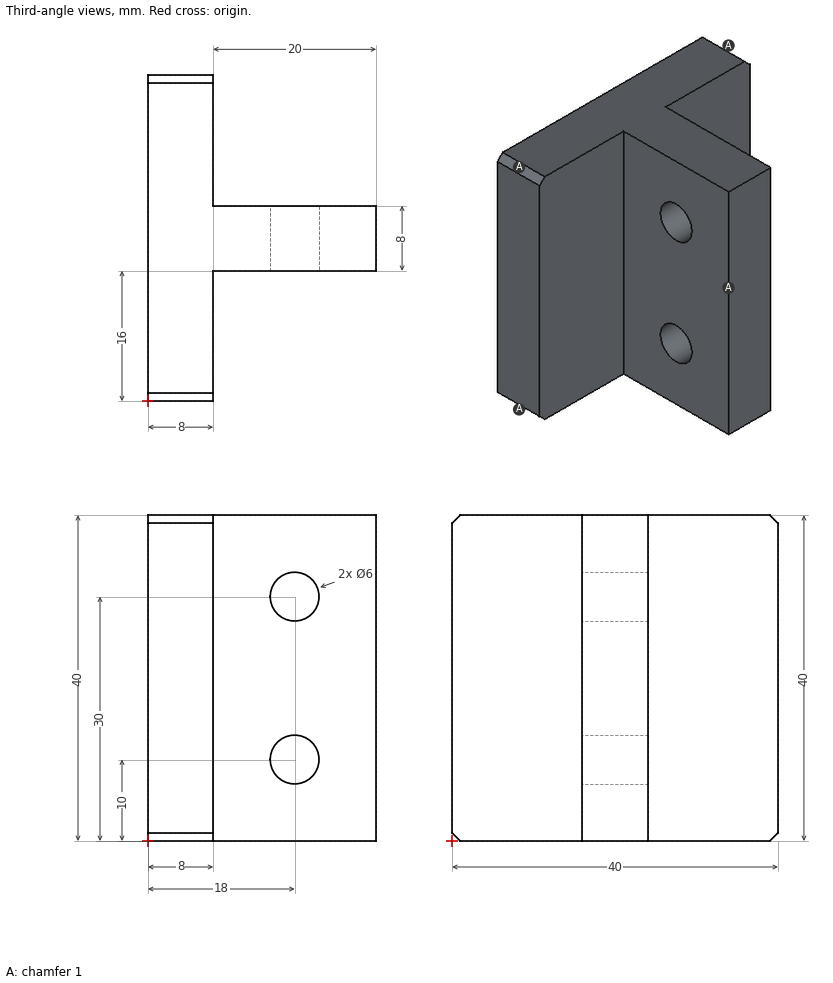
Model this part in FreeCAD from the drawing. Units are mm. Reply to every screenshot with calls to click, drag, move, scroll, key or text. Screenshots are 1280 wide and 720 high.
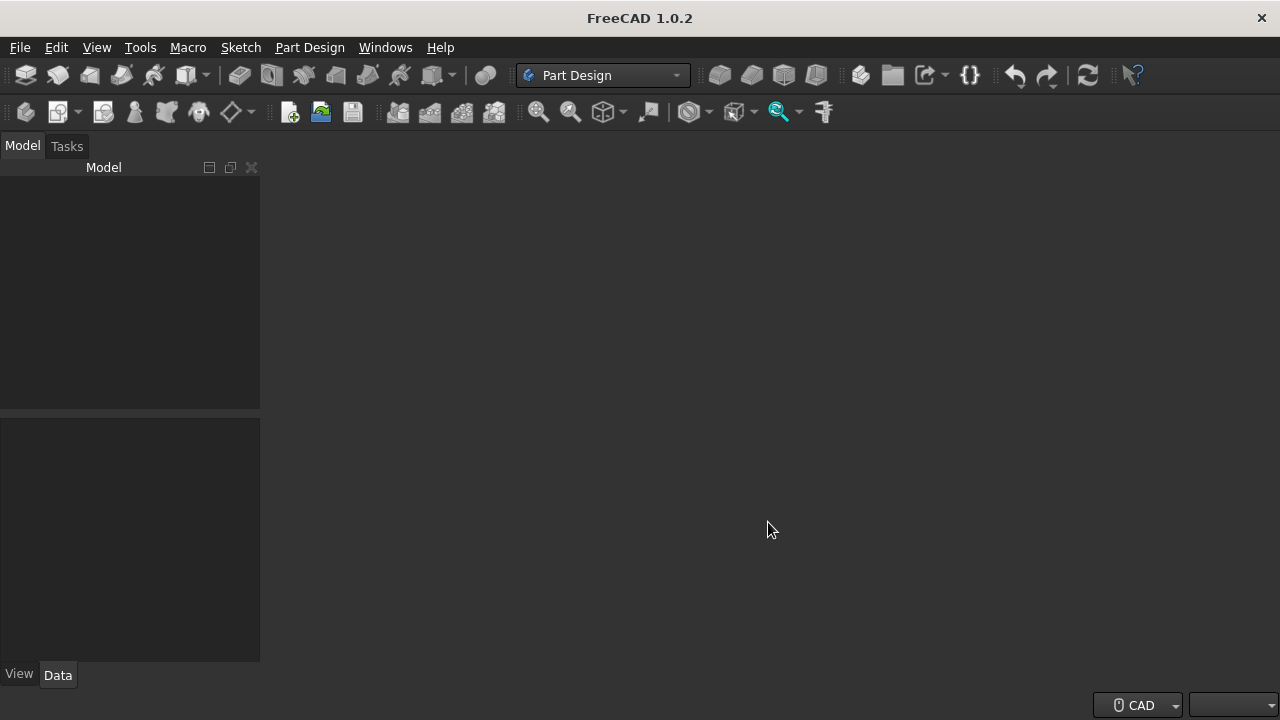
click(290, 112)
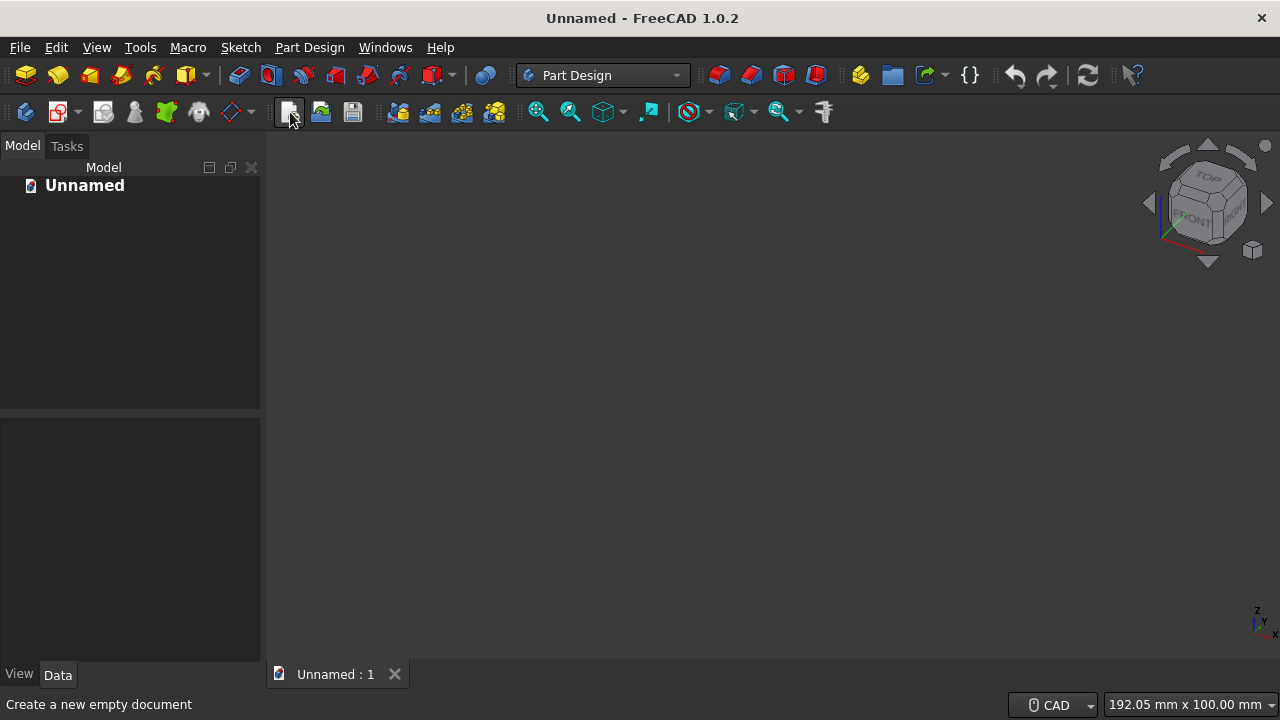
click(58, 112)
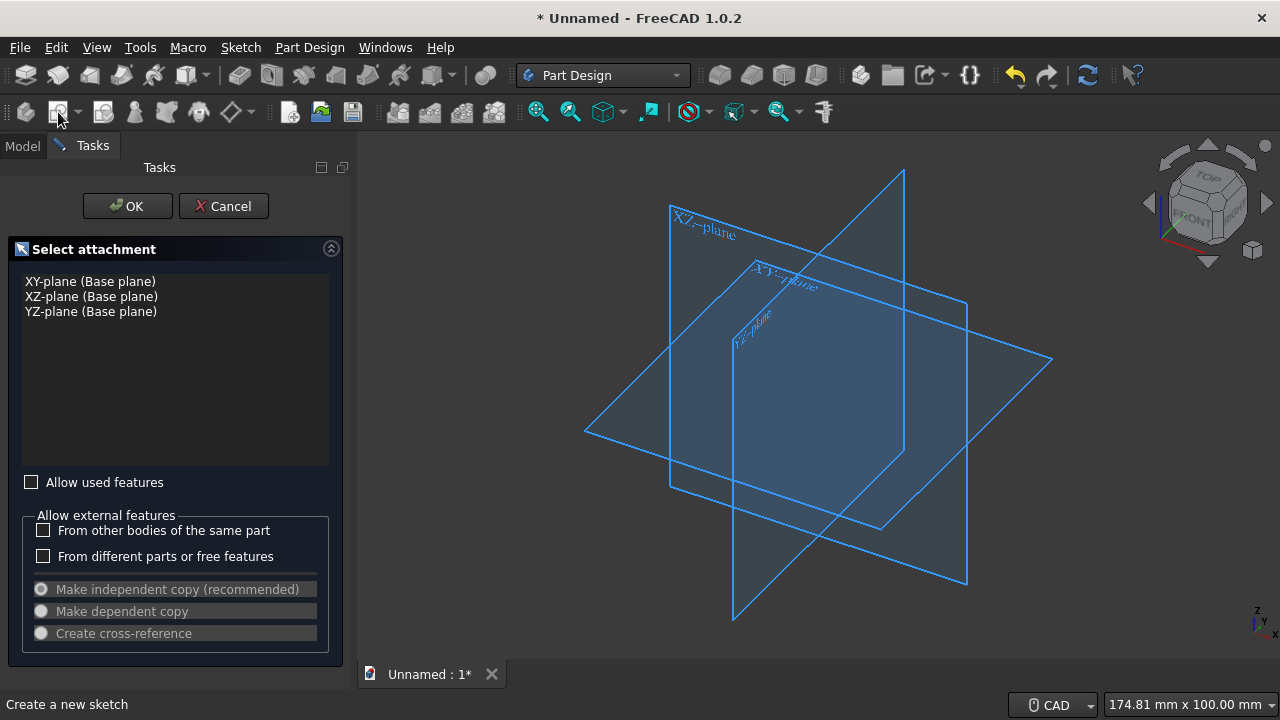
click(82, 296)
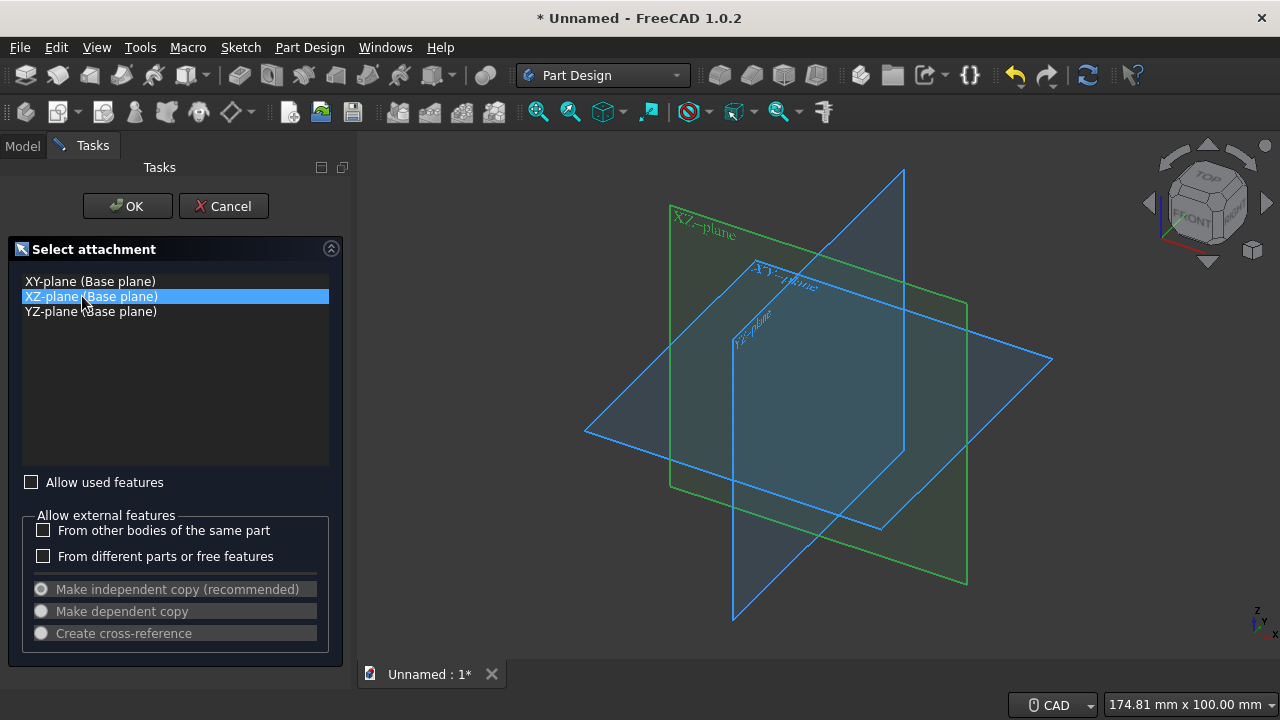
click(128, 206)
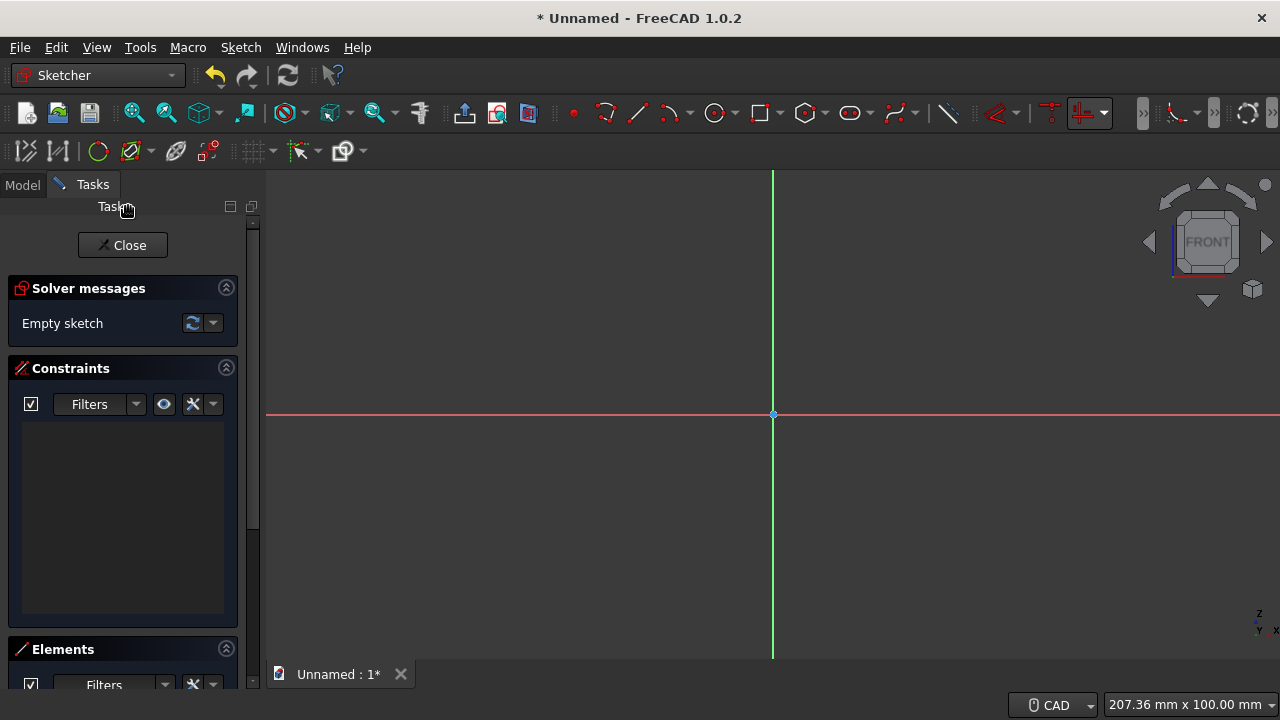
scroll(972, 198, up, 2)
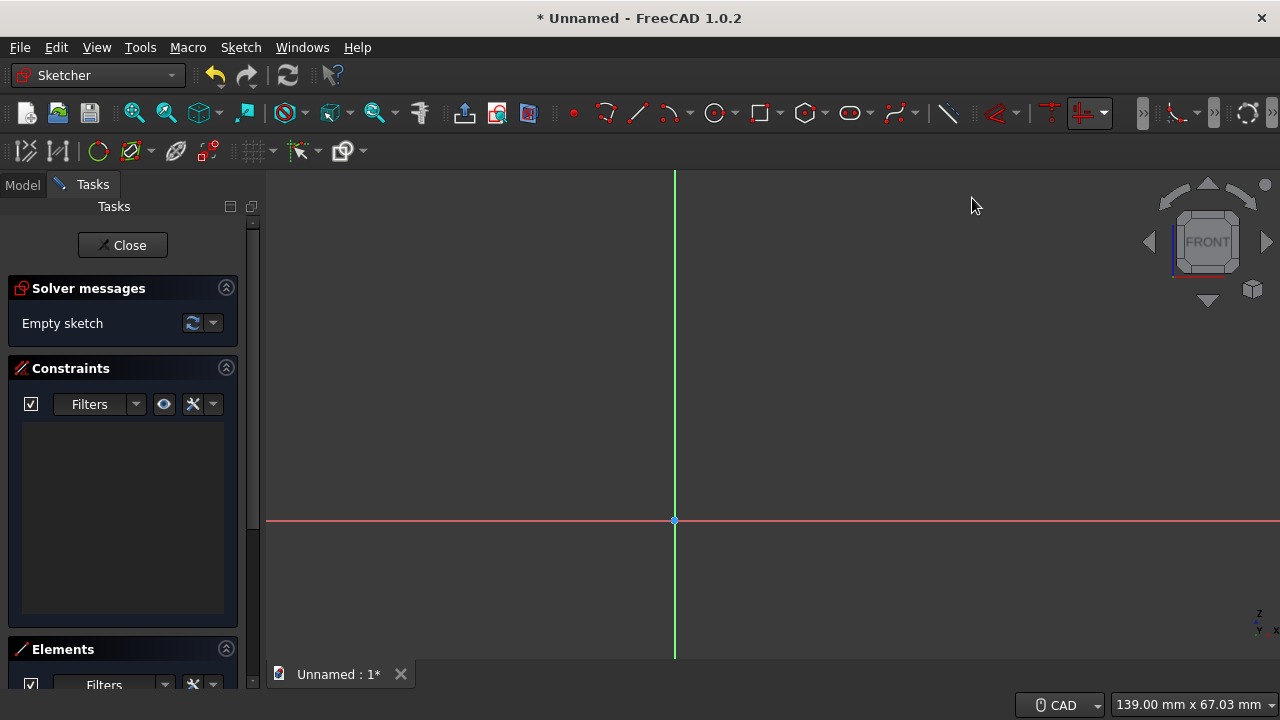
click(760, 114)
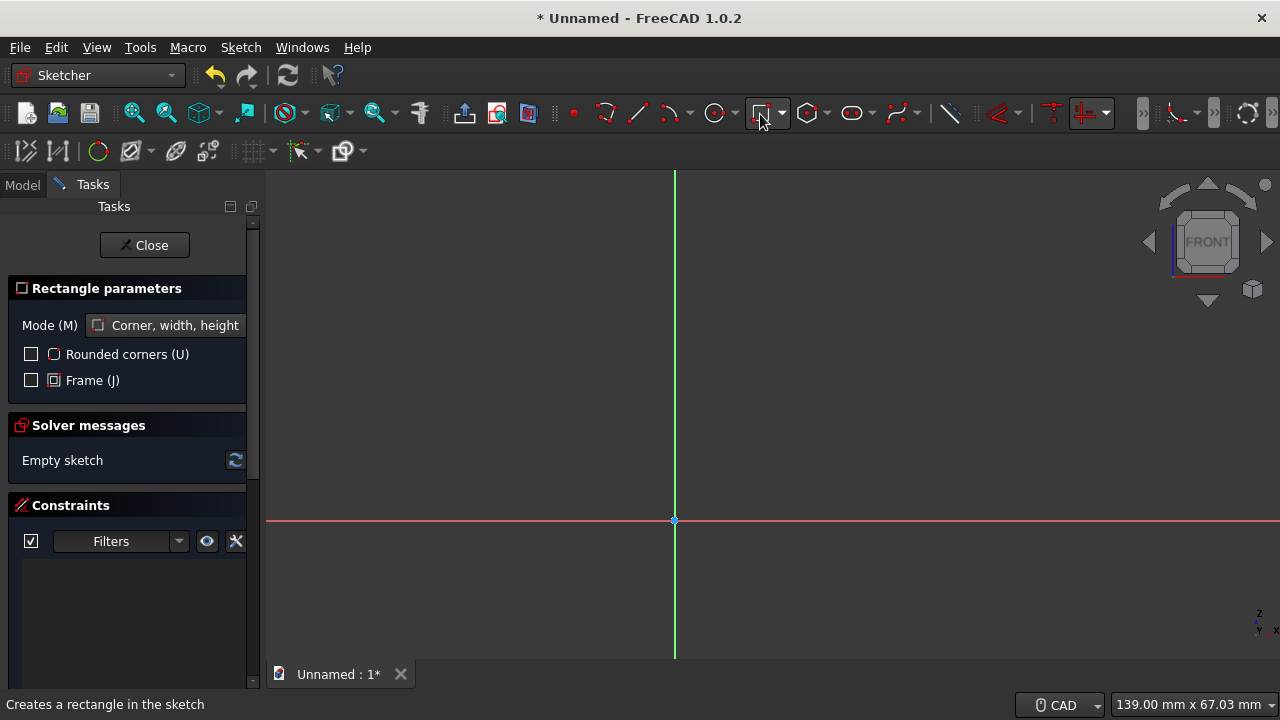
click(675, 521)
click(733, 229)
key(Escape)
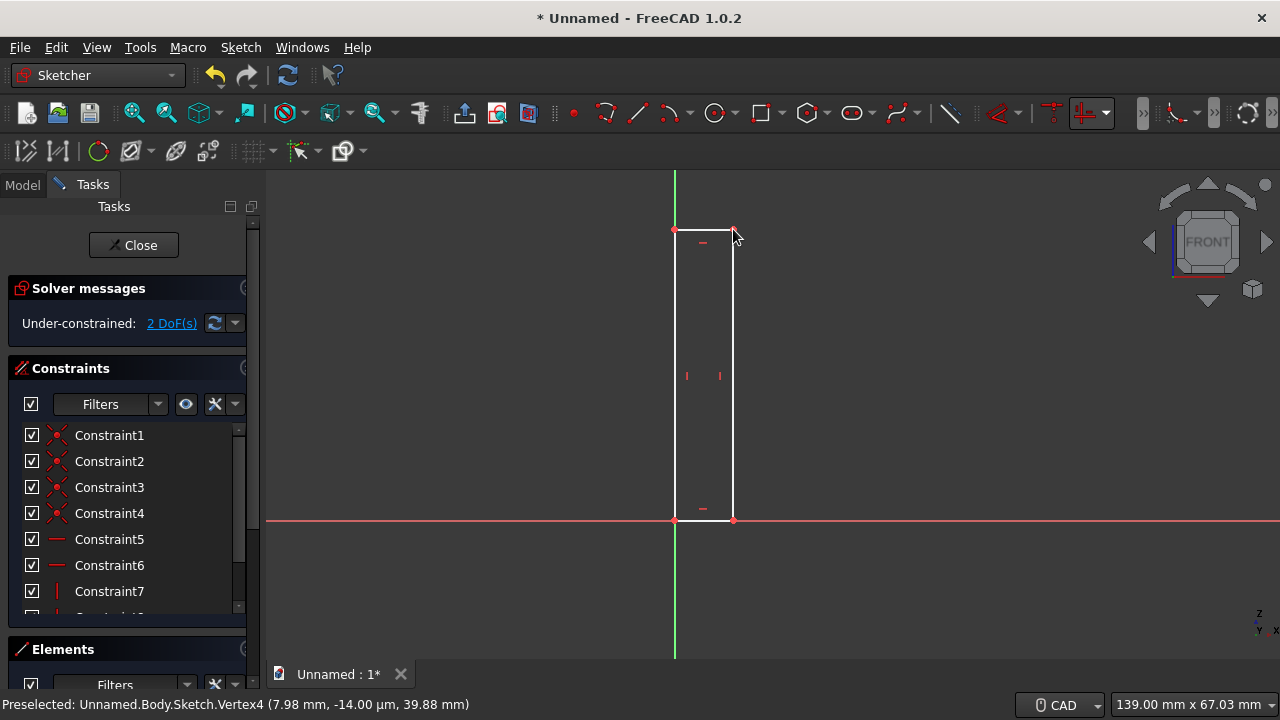
key(d)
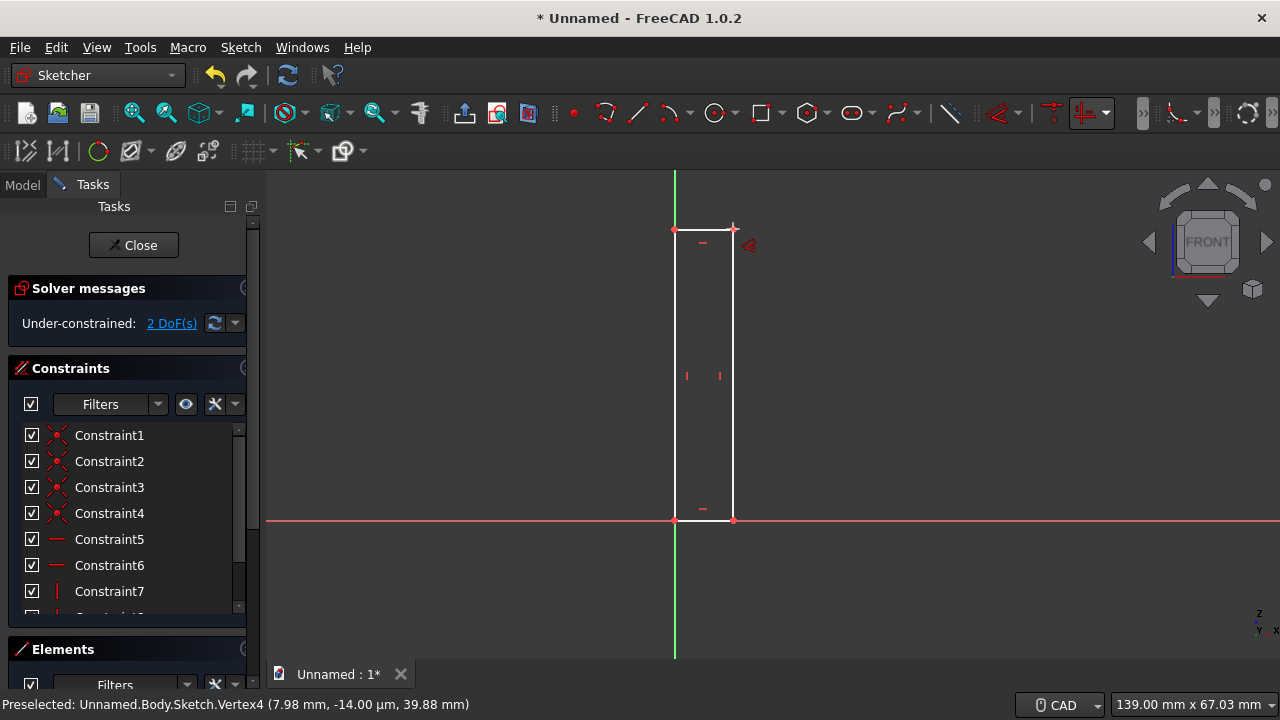
click(692, 521)
click(704, 555)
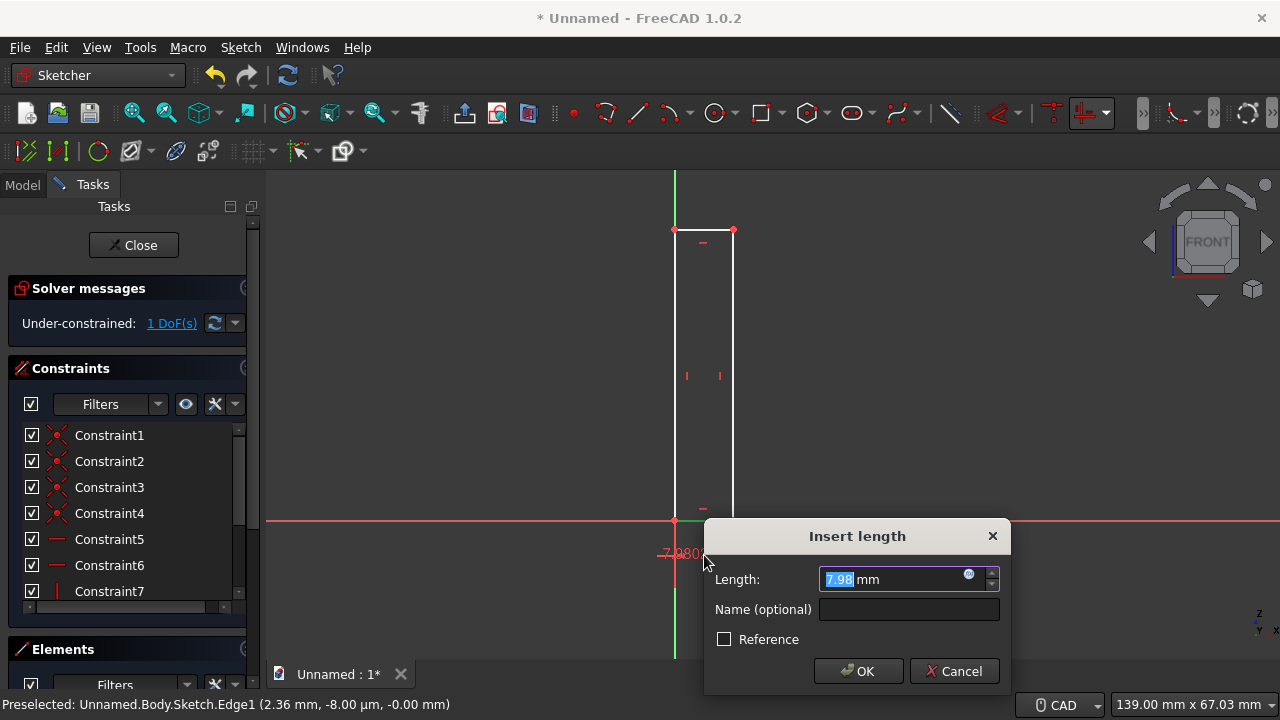
text(8)
key(Return)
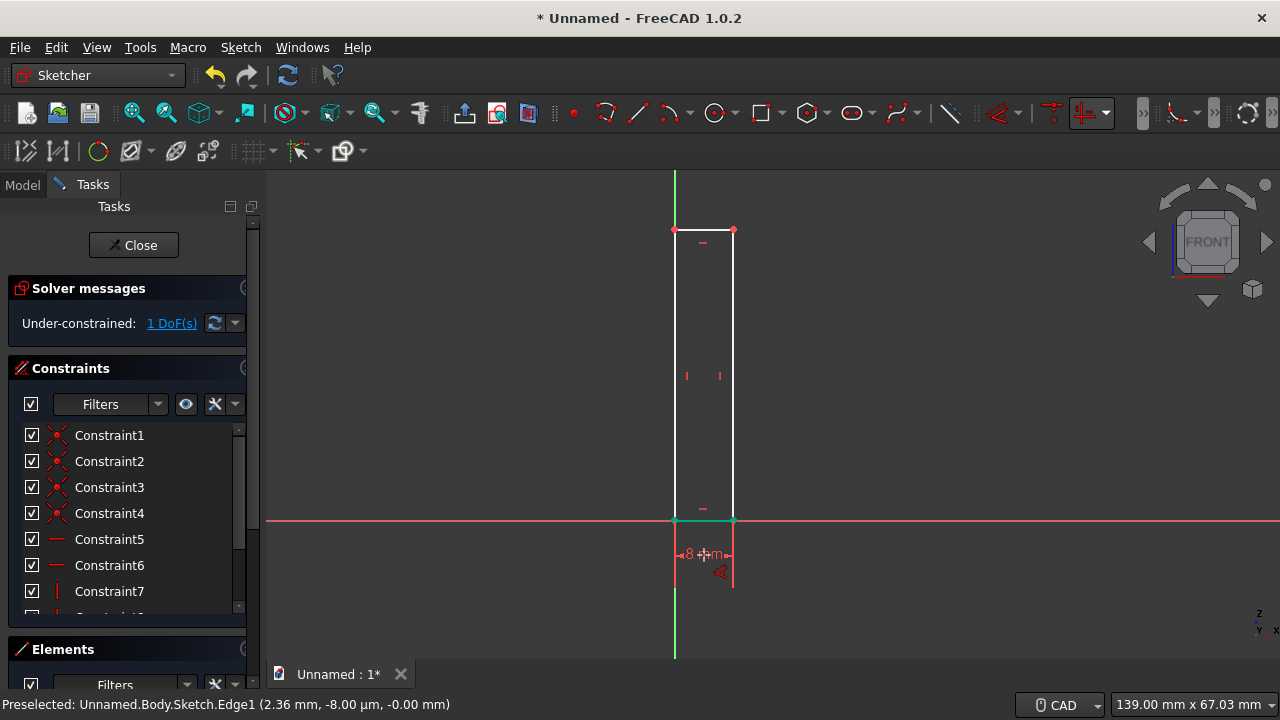
click(733, 434)
click(767, 375)